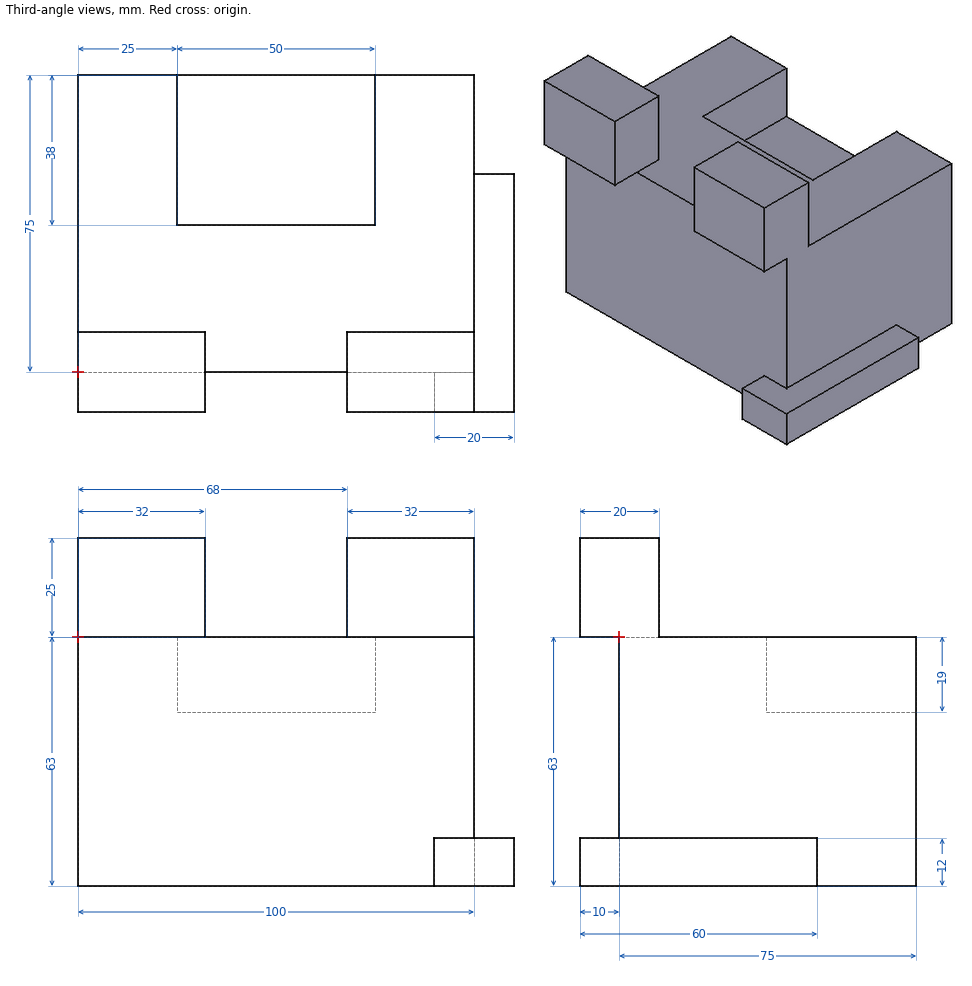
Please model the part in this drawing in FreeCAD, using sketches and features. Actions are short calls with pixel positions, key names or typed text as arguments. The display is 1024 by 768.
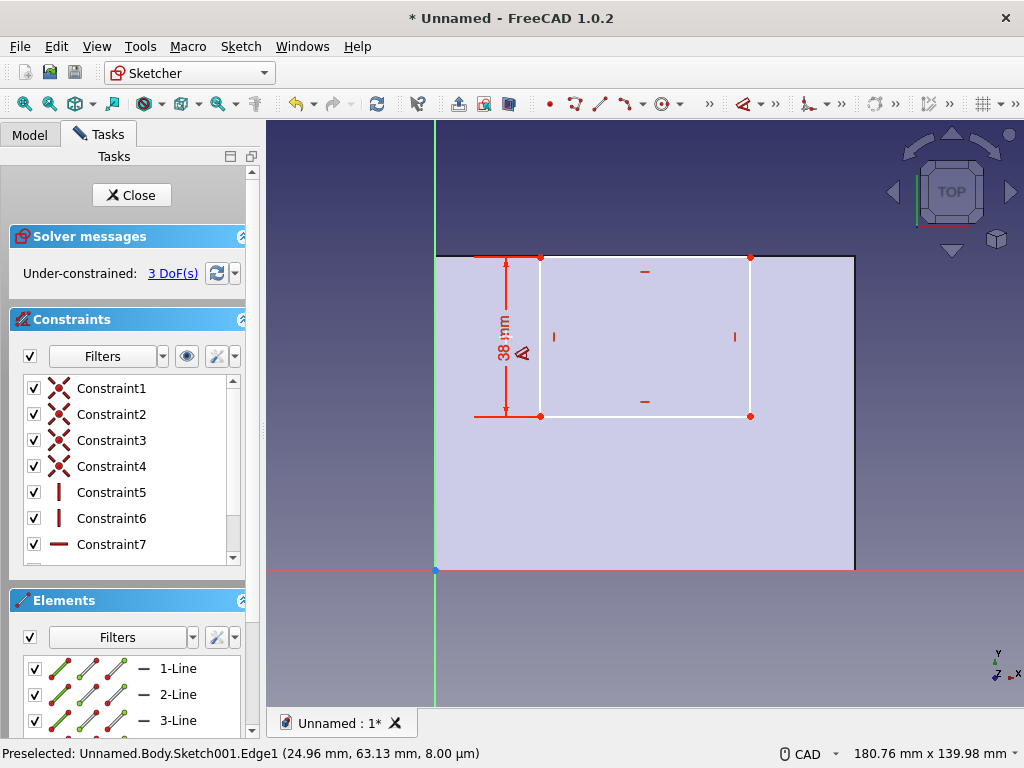
click(603, 417)
click(645, 451)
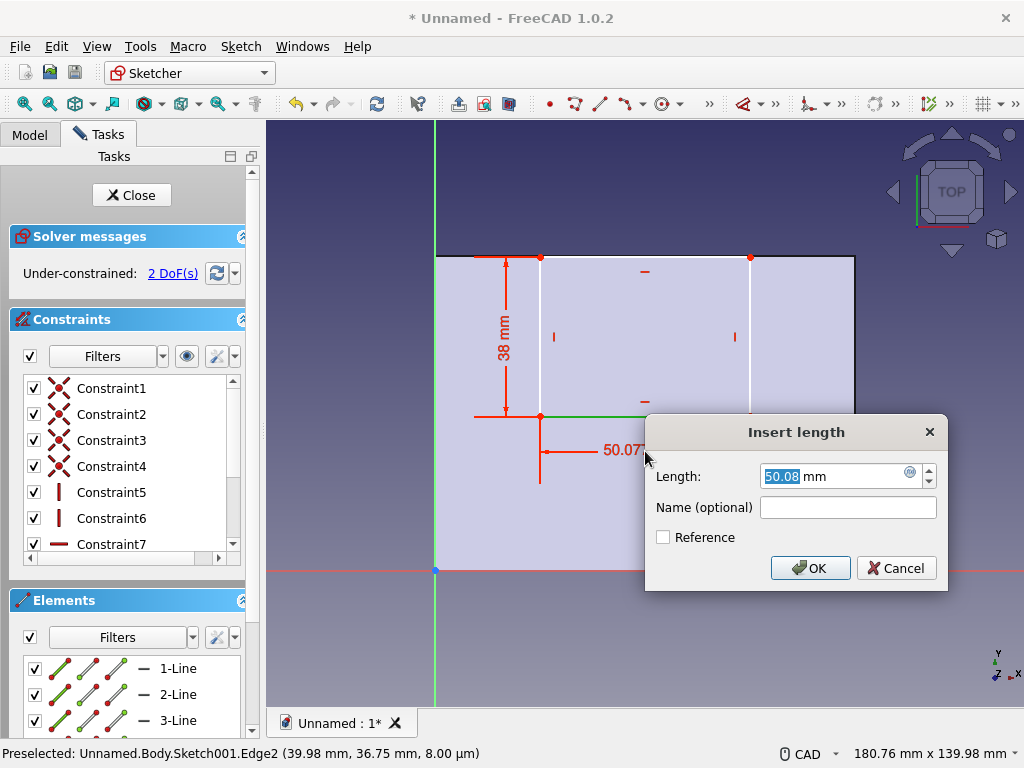
text(50)
key(Return)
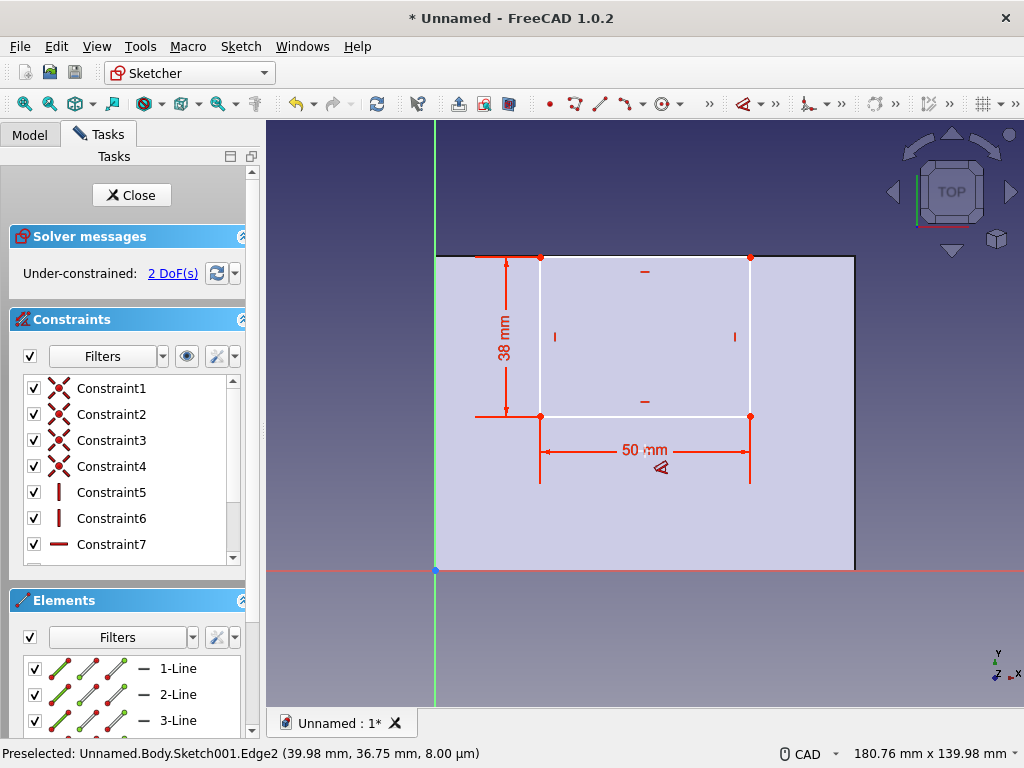
click(540, 257)
click(488, 605)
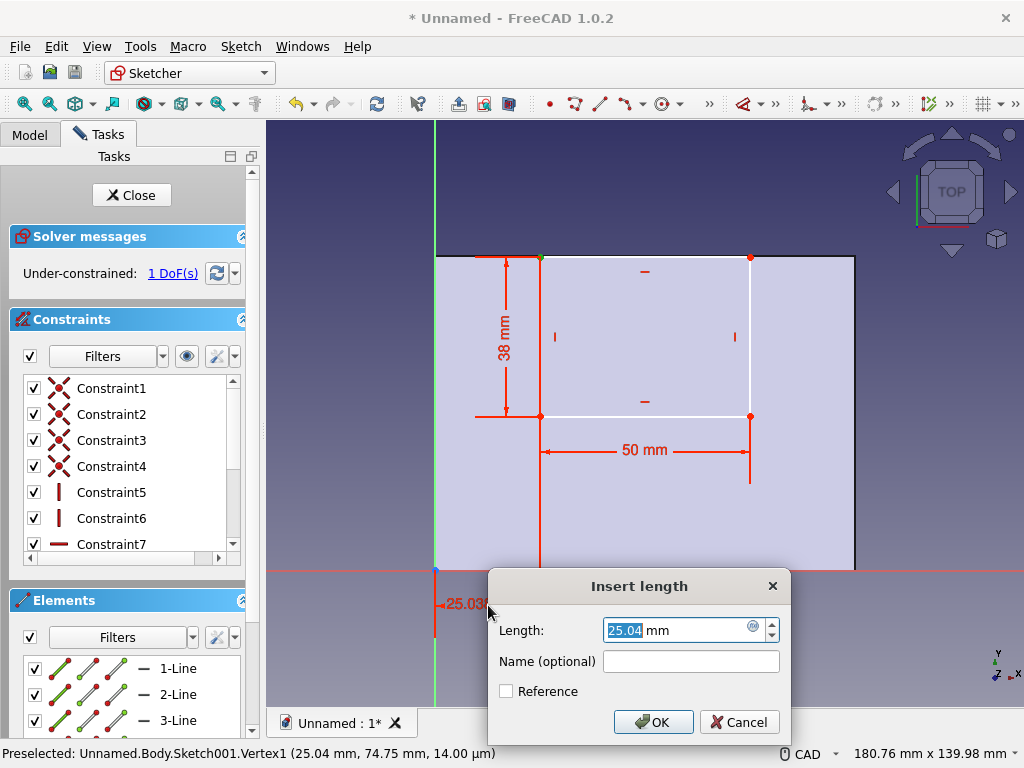
text(25)
key(Return)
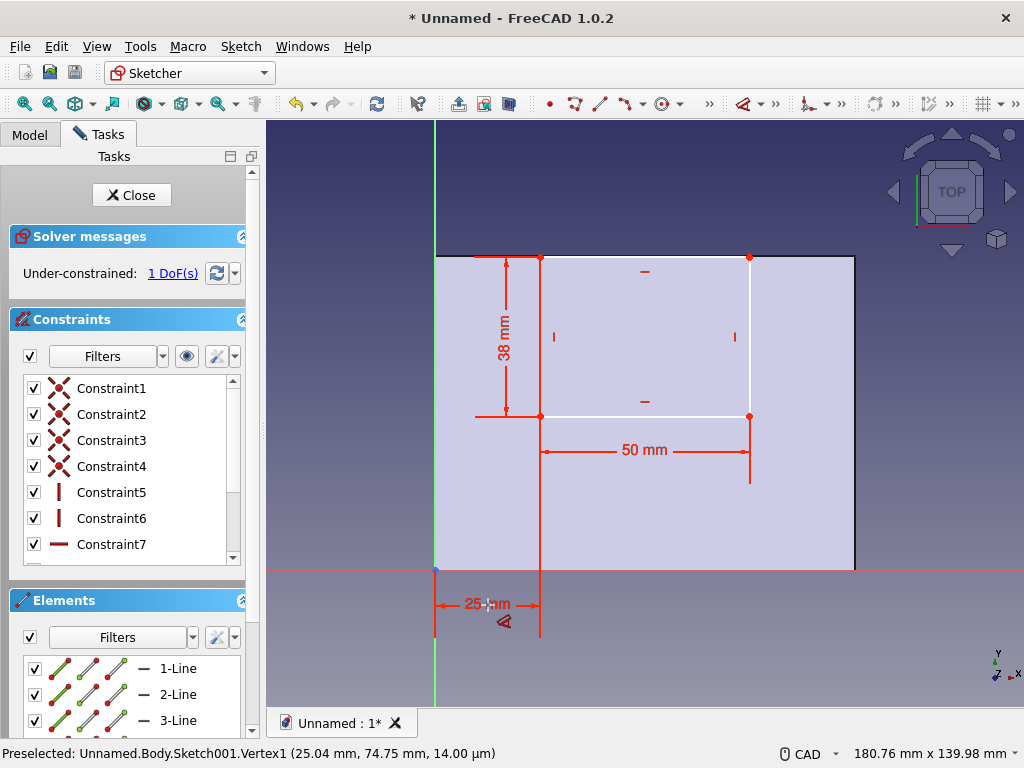
click(540, 257)
click(401, 414)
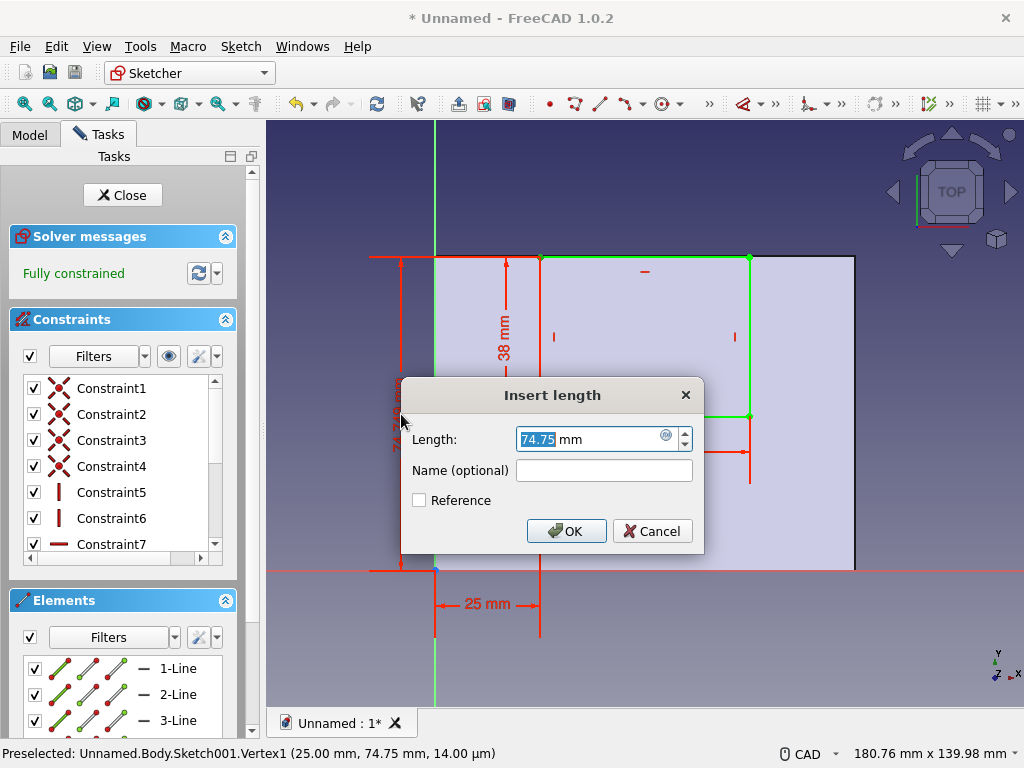
text(75)
key(Return)
key(Escape)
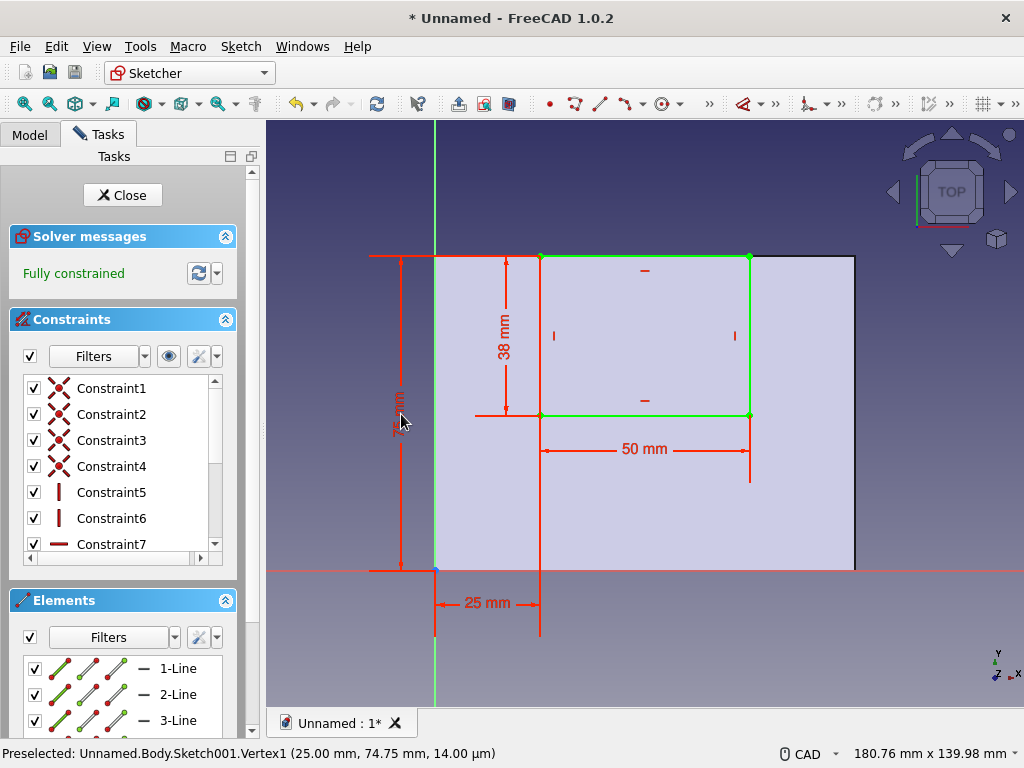
click(123, 195)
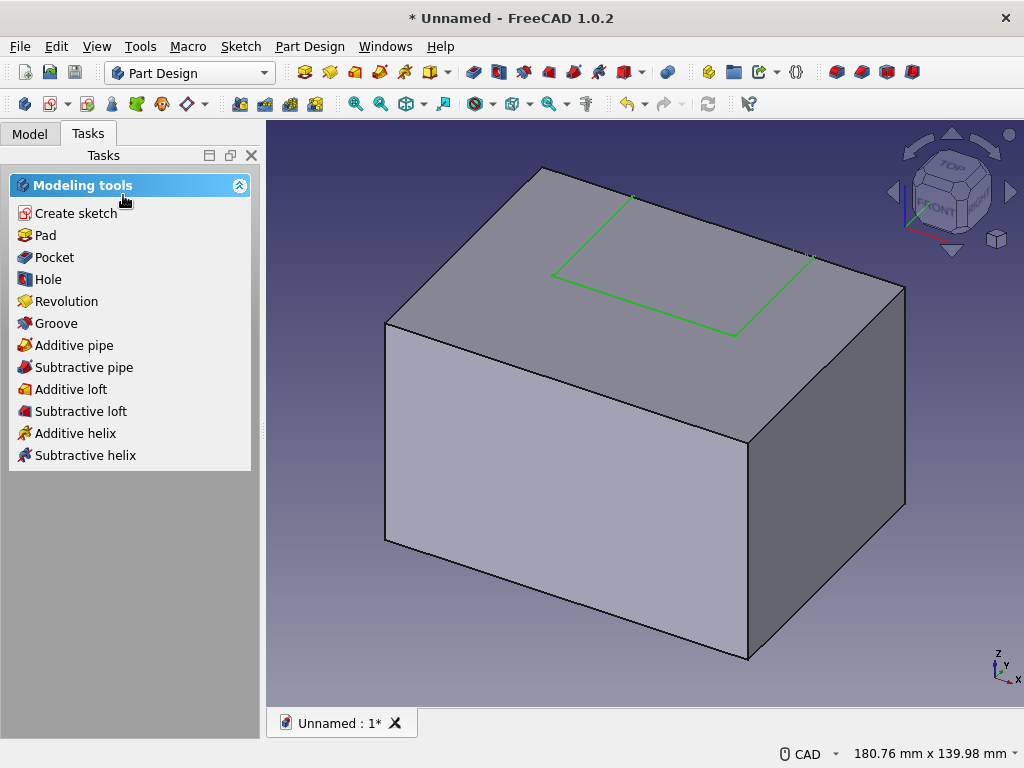
click(474, 72)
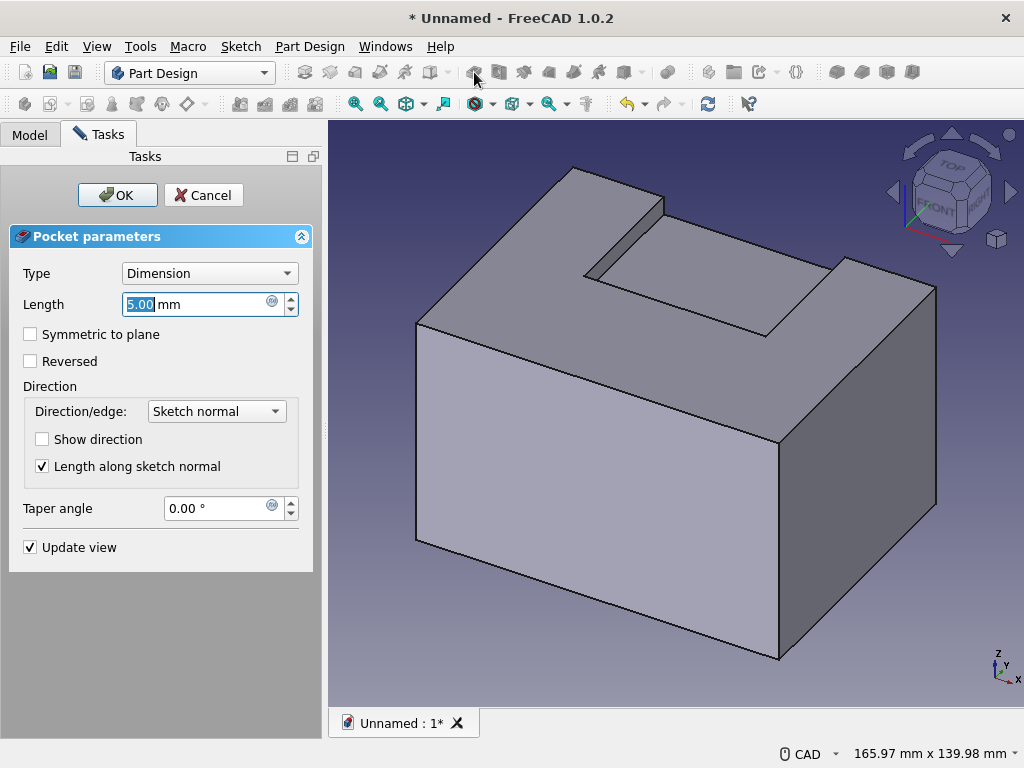
text(19)
key(Tab)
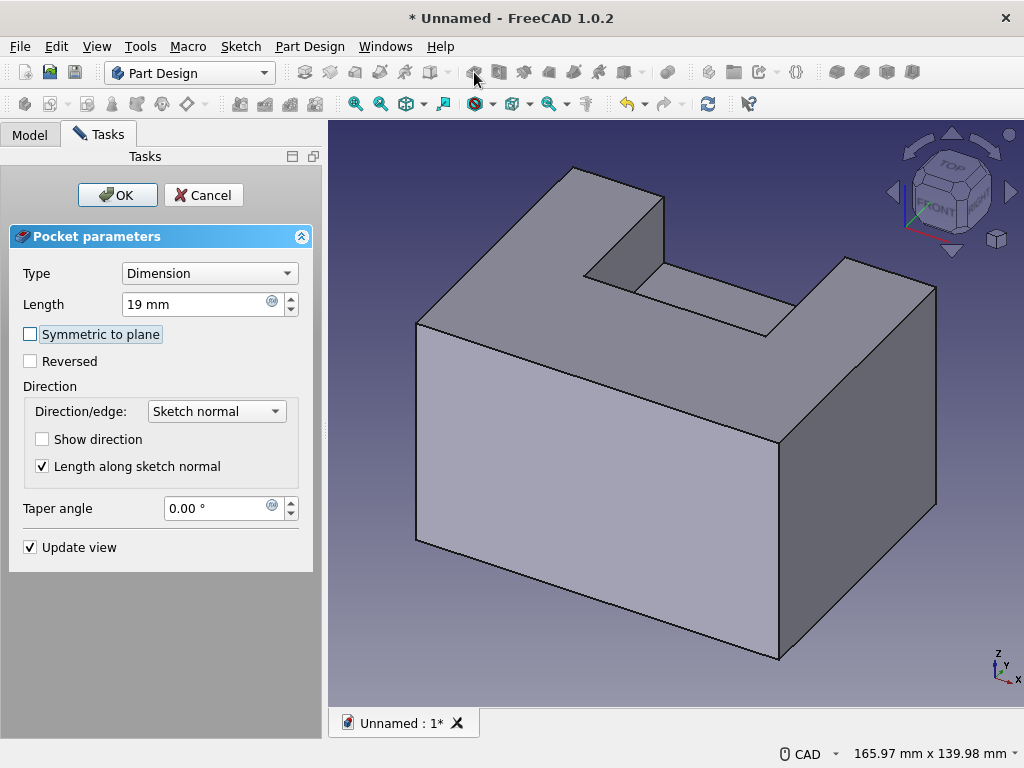
click(118, 195)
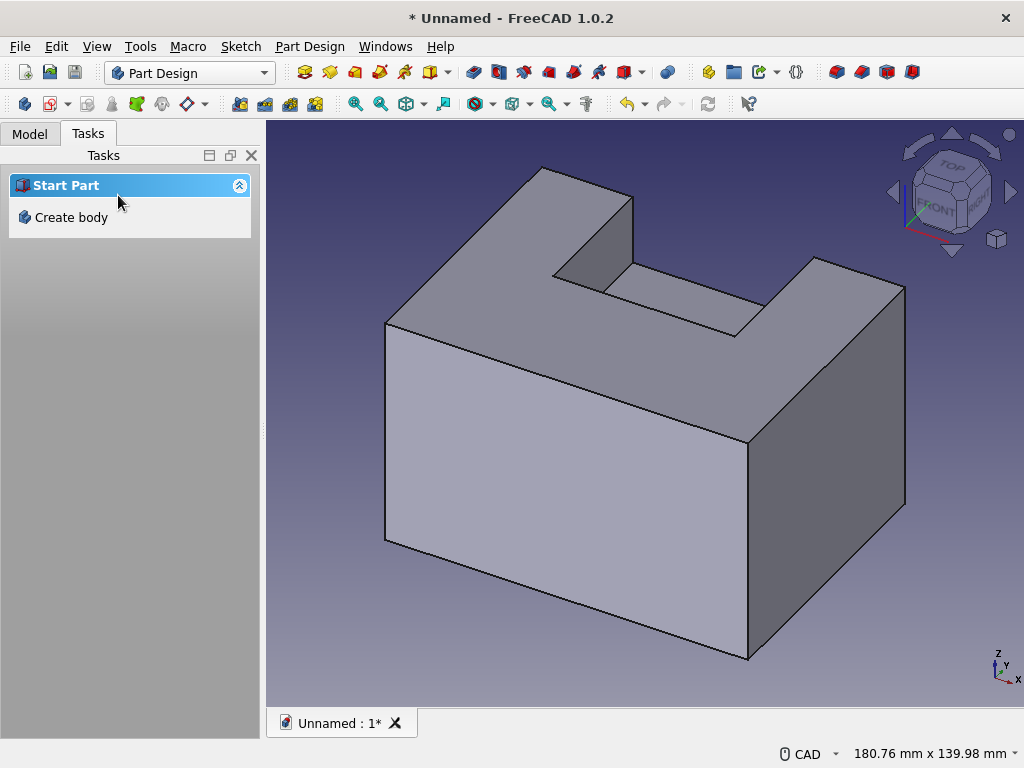
click(50, 104)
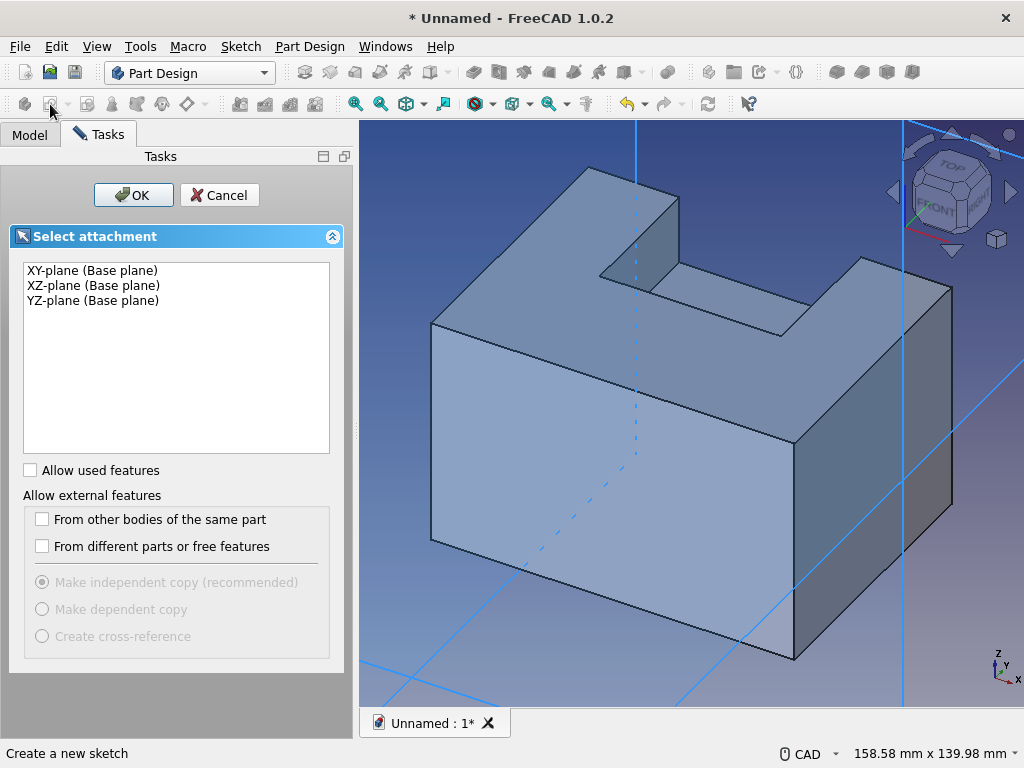
click(84, 286)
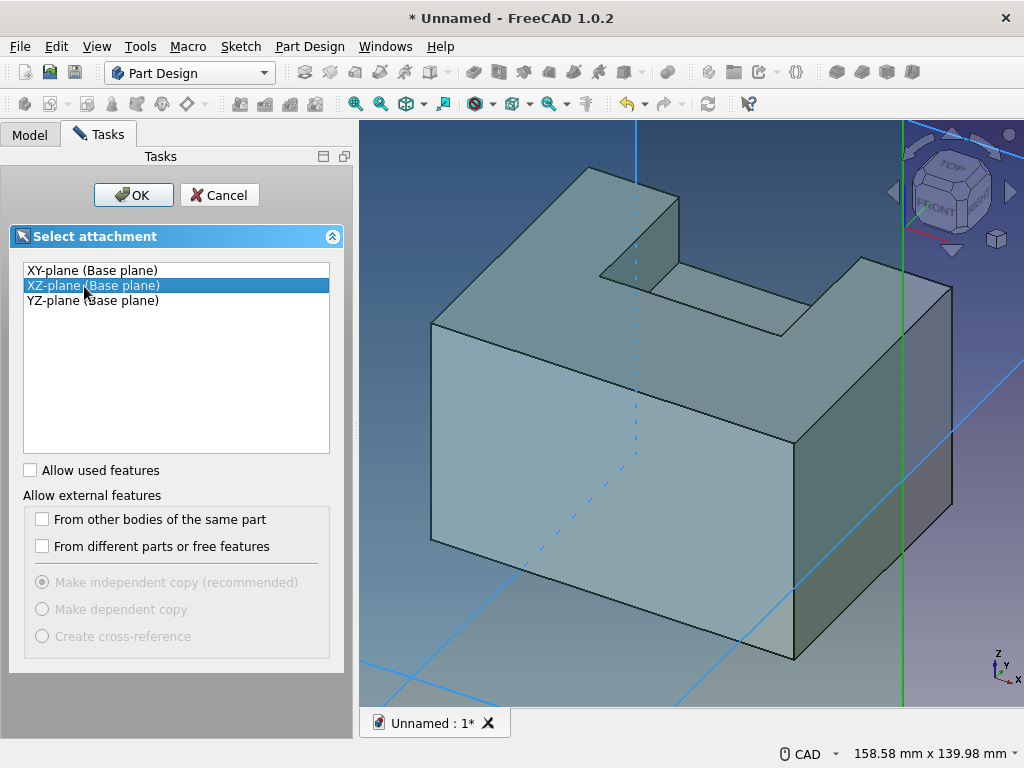
click(134, 195)